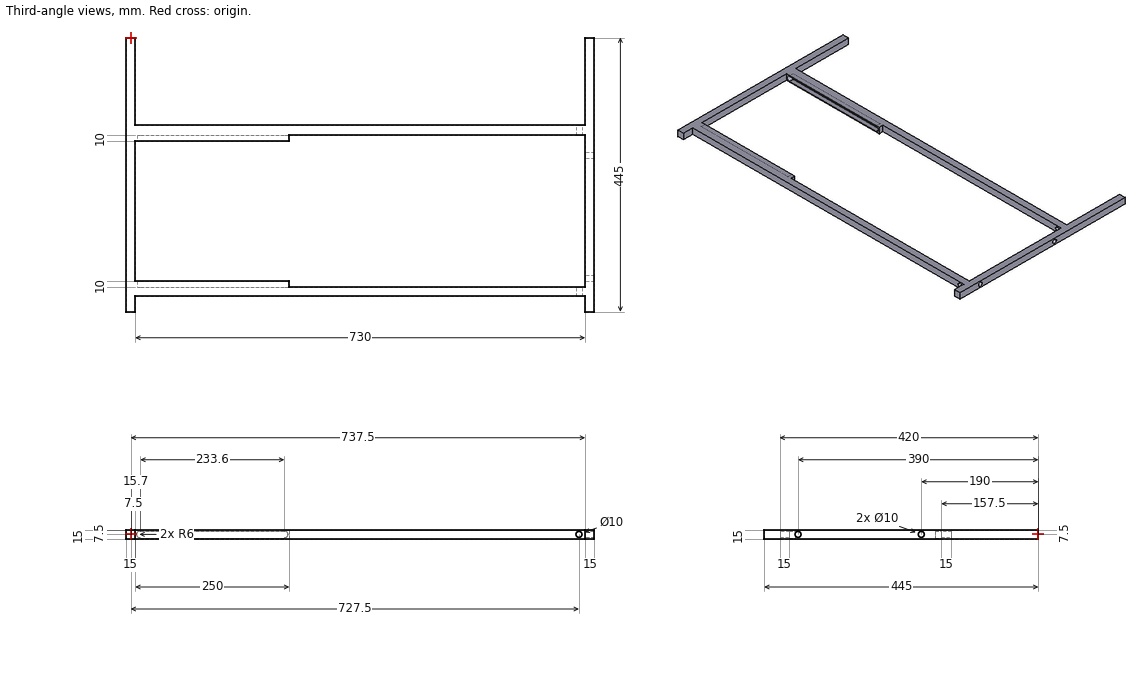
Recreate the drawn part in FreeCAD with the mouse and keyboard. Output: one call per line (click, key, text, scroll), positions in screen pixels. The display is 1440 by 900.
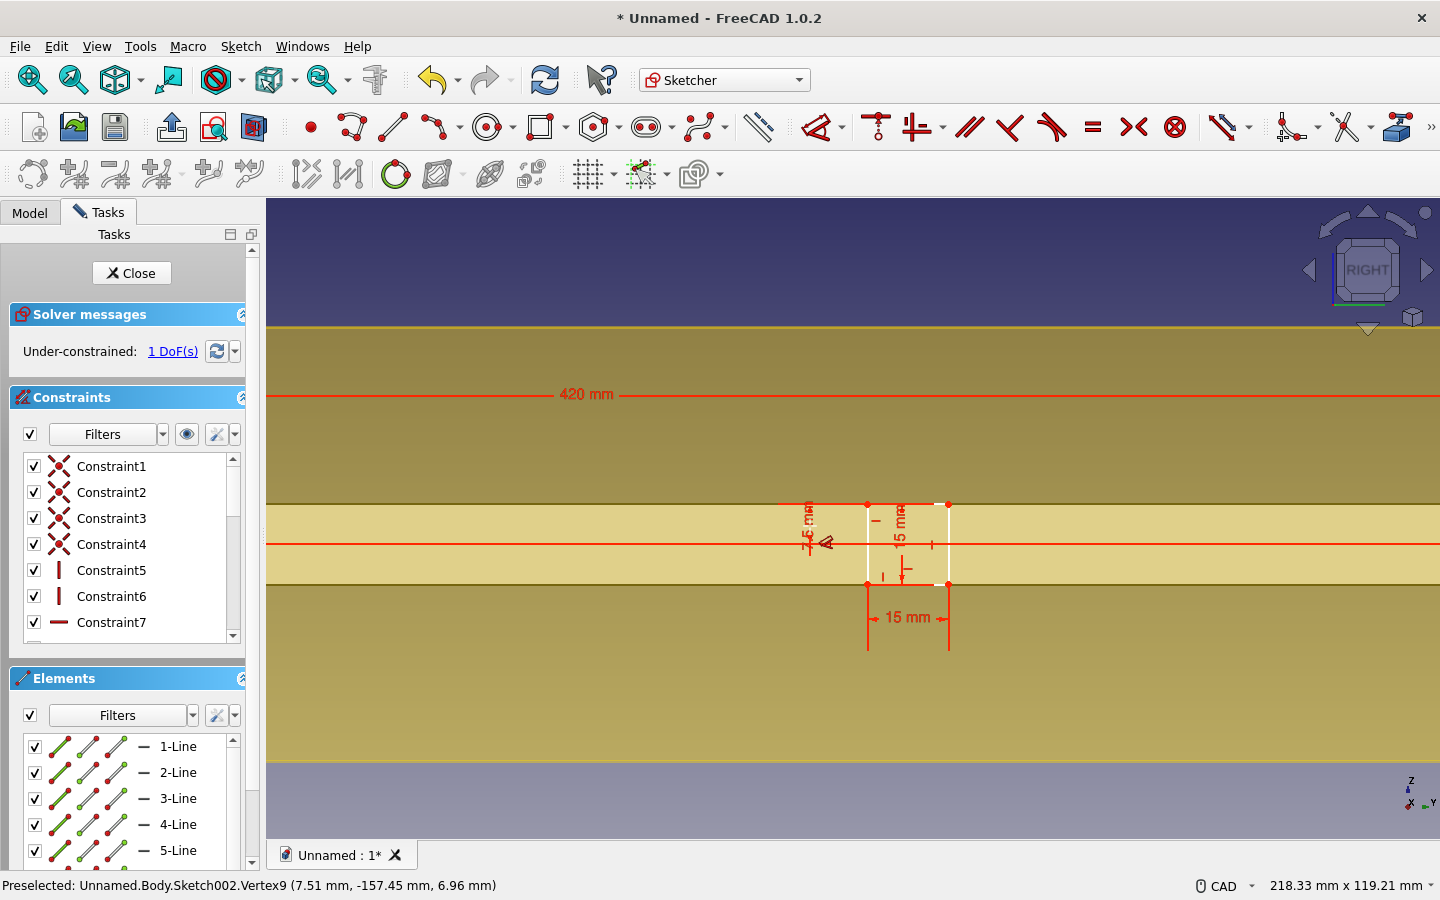
click(868, 504)
click(1071, 470)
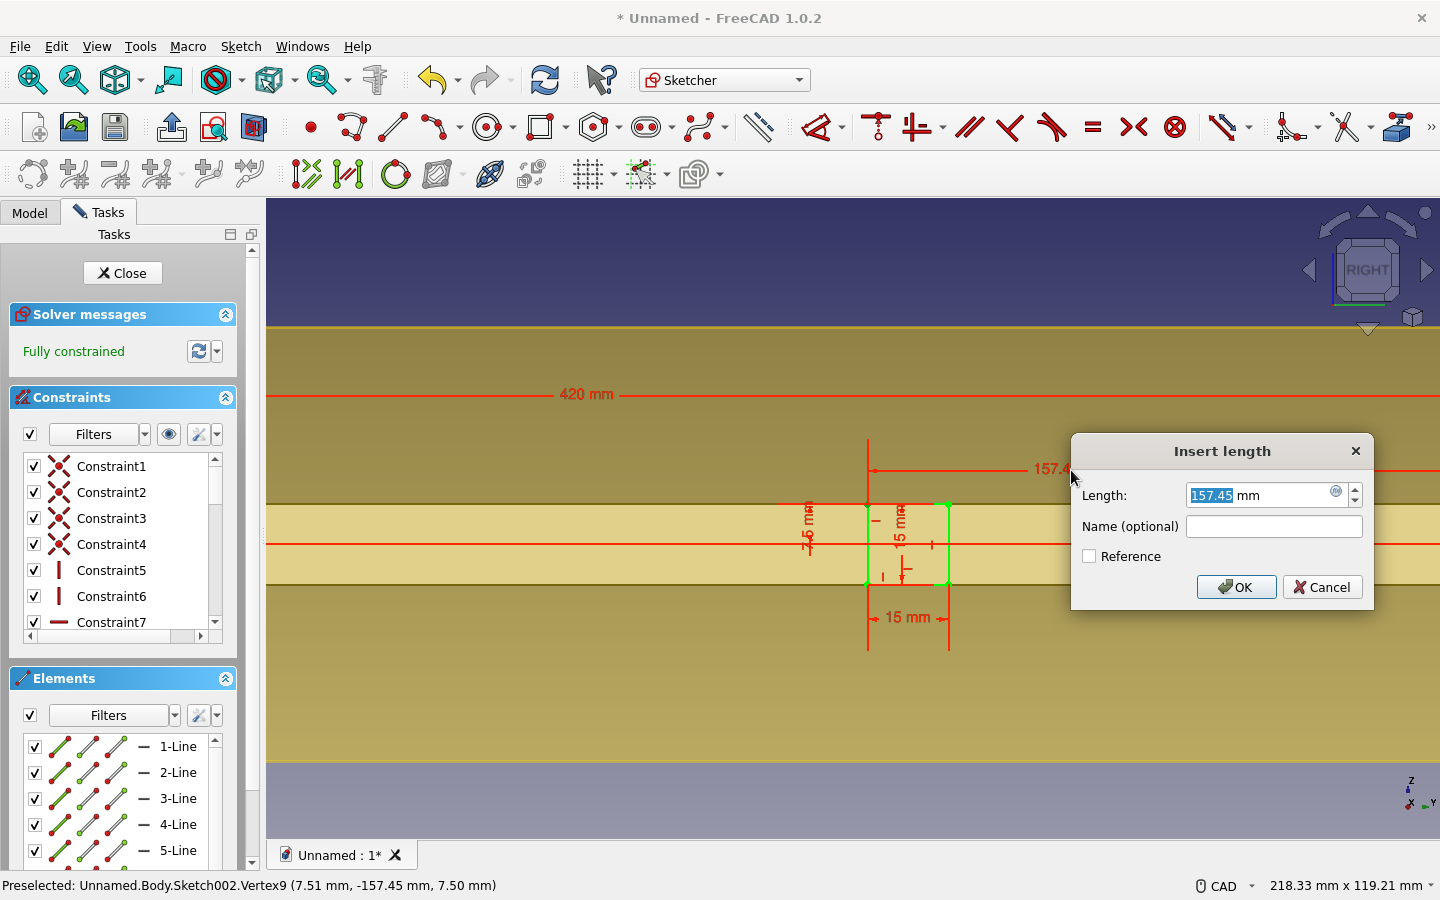
text(157.5)
key(Return)
key(Escape)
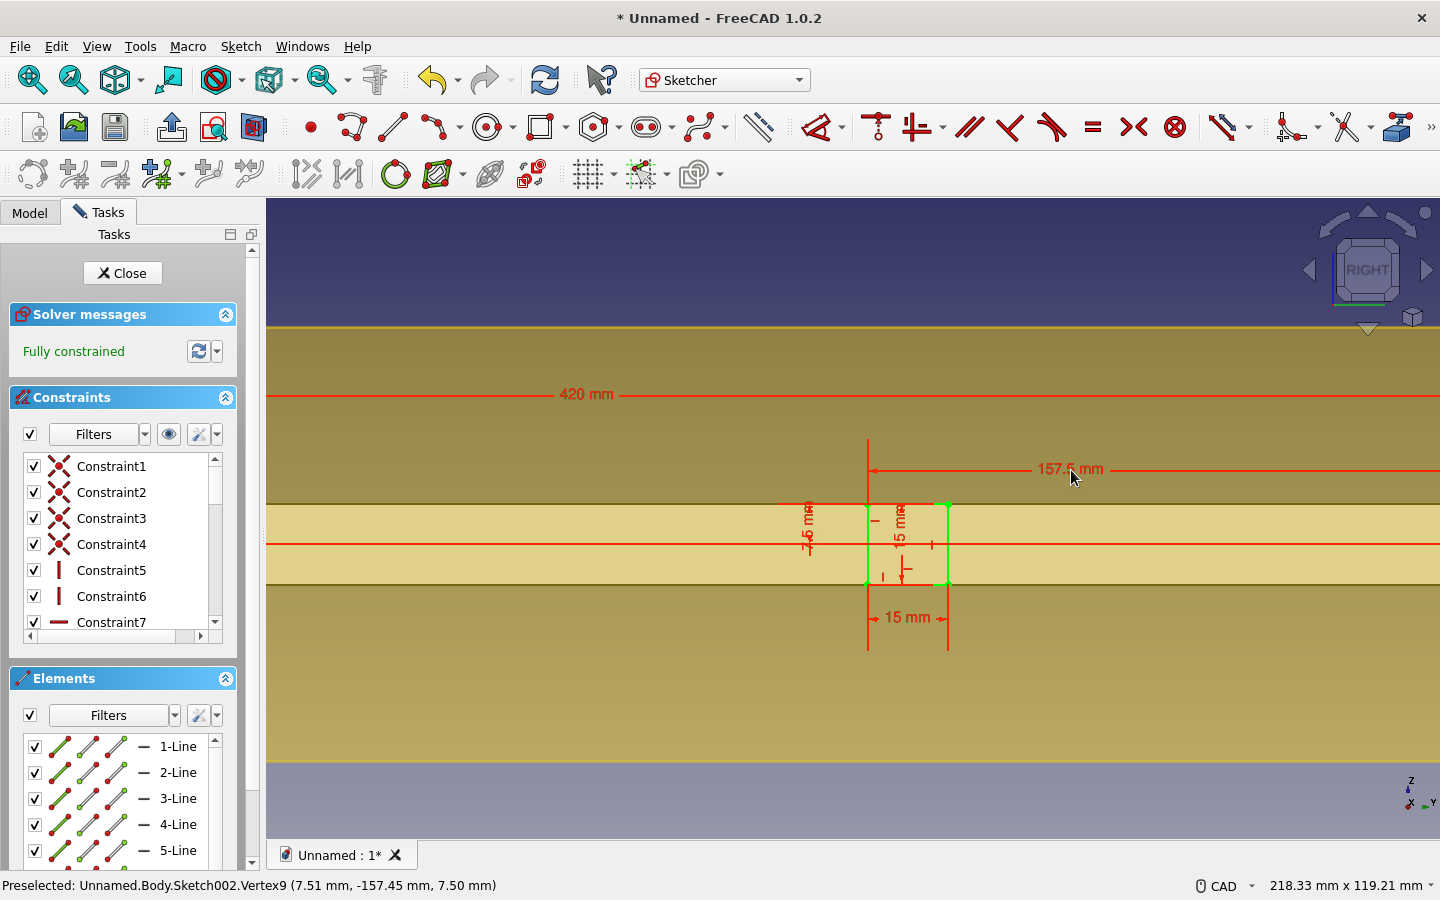
click(123, 273)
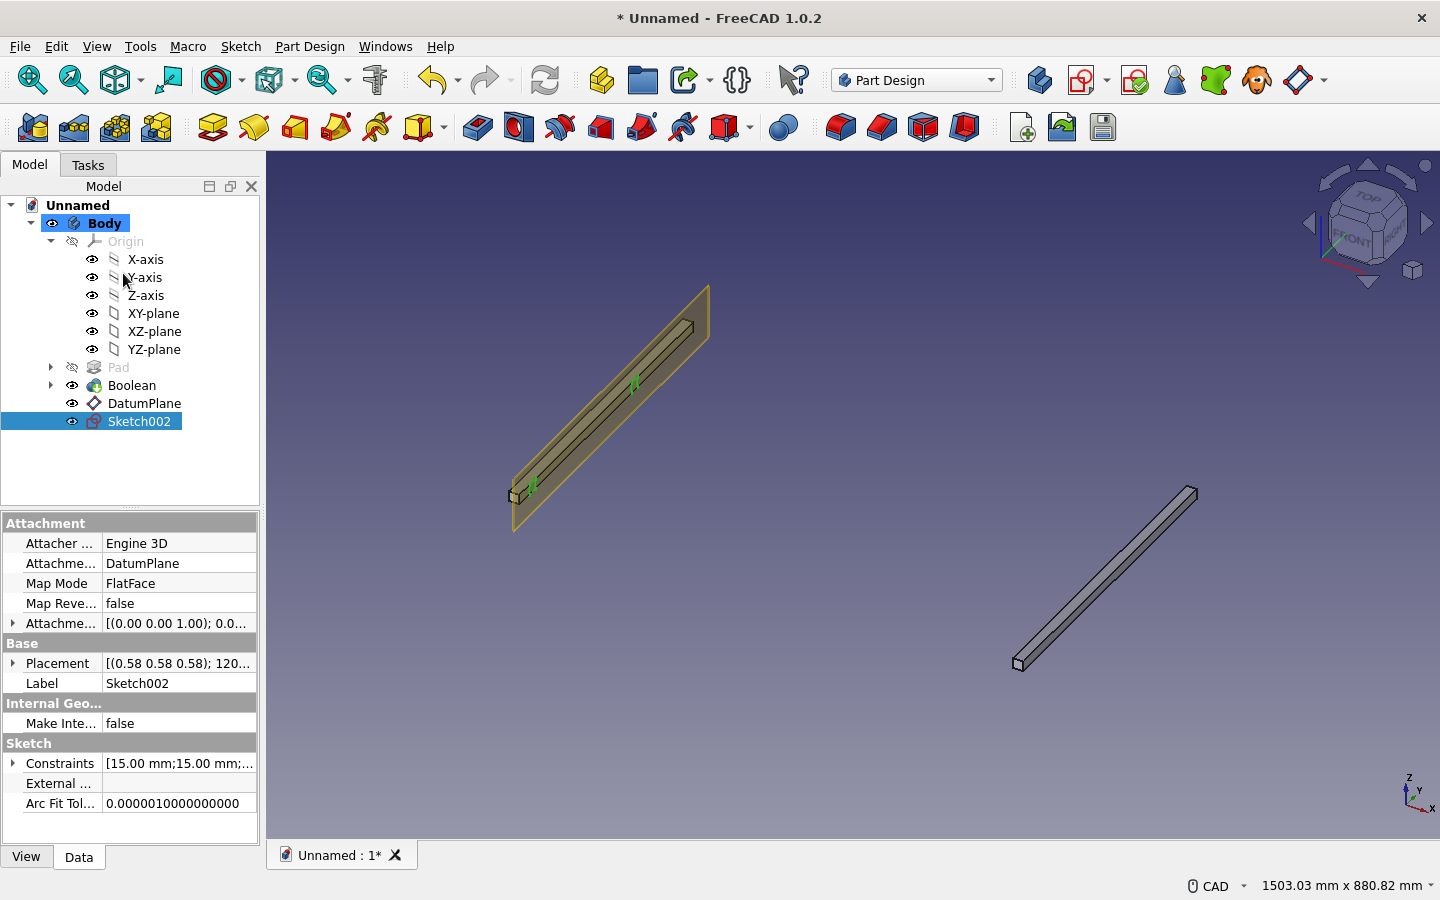
click(213, 128)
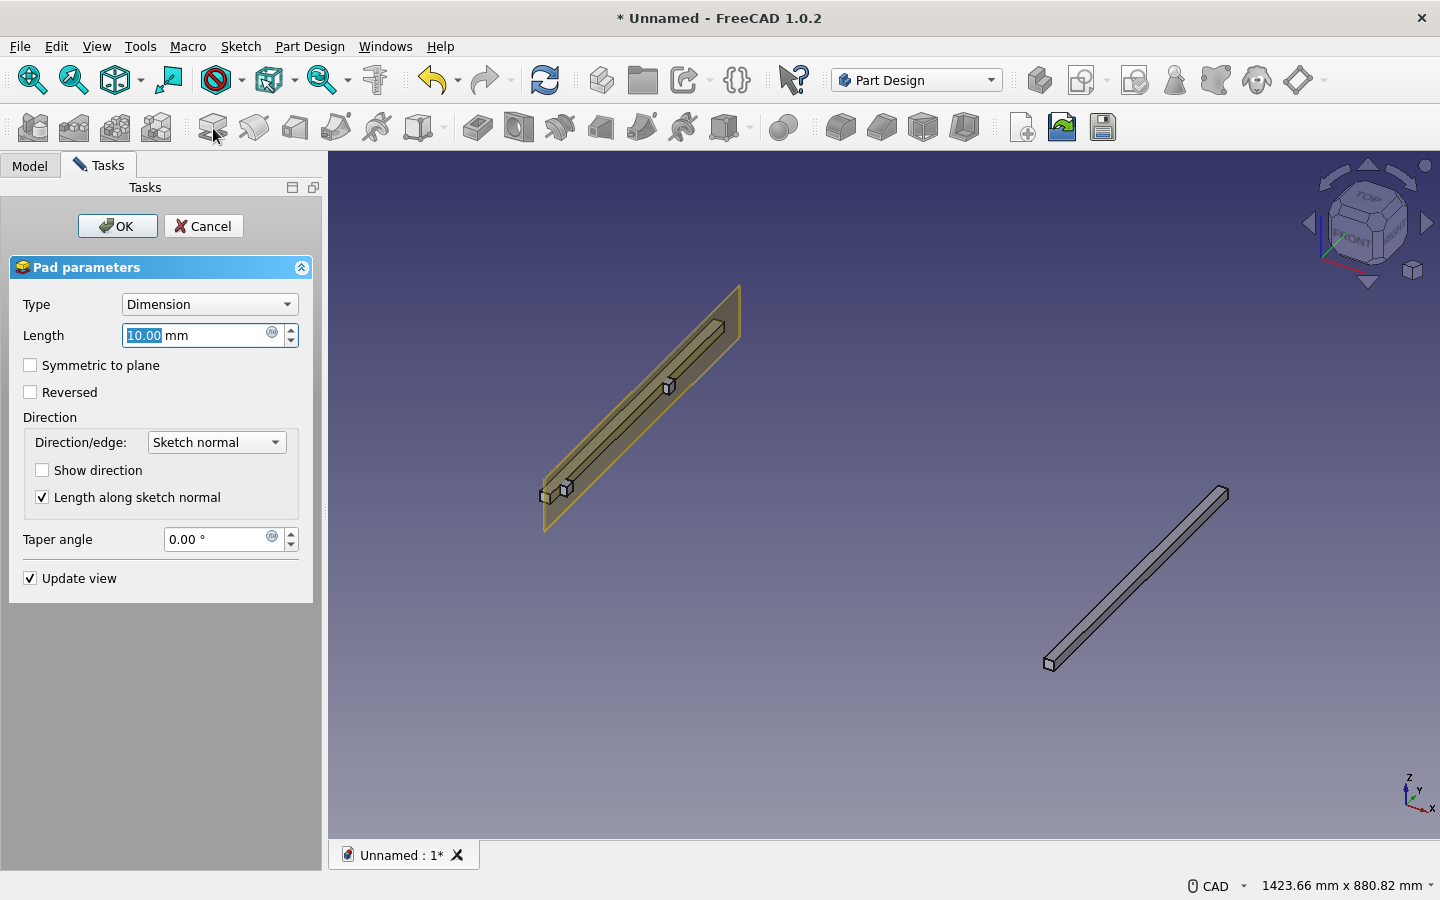
text(730)
key(Tab)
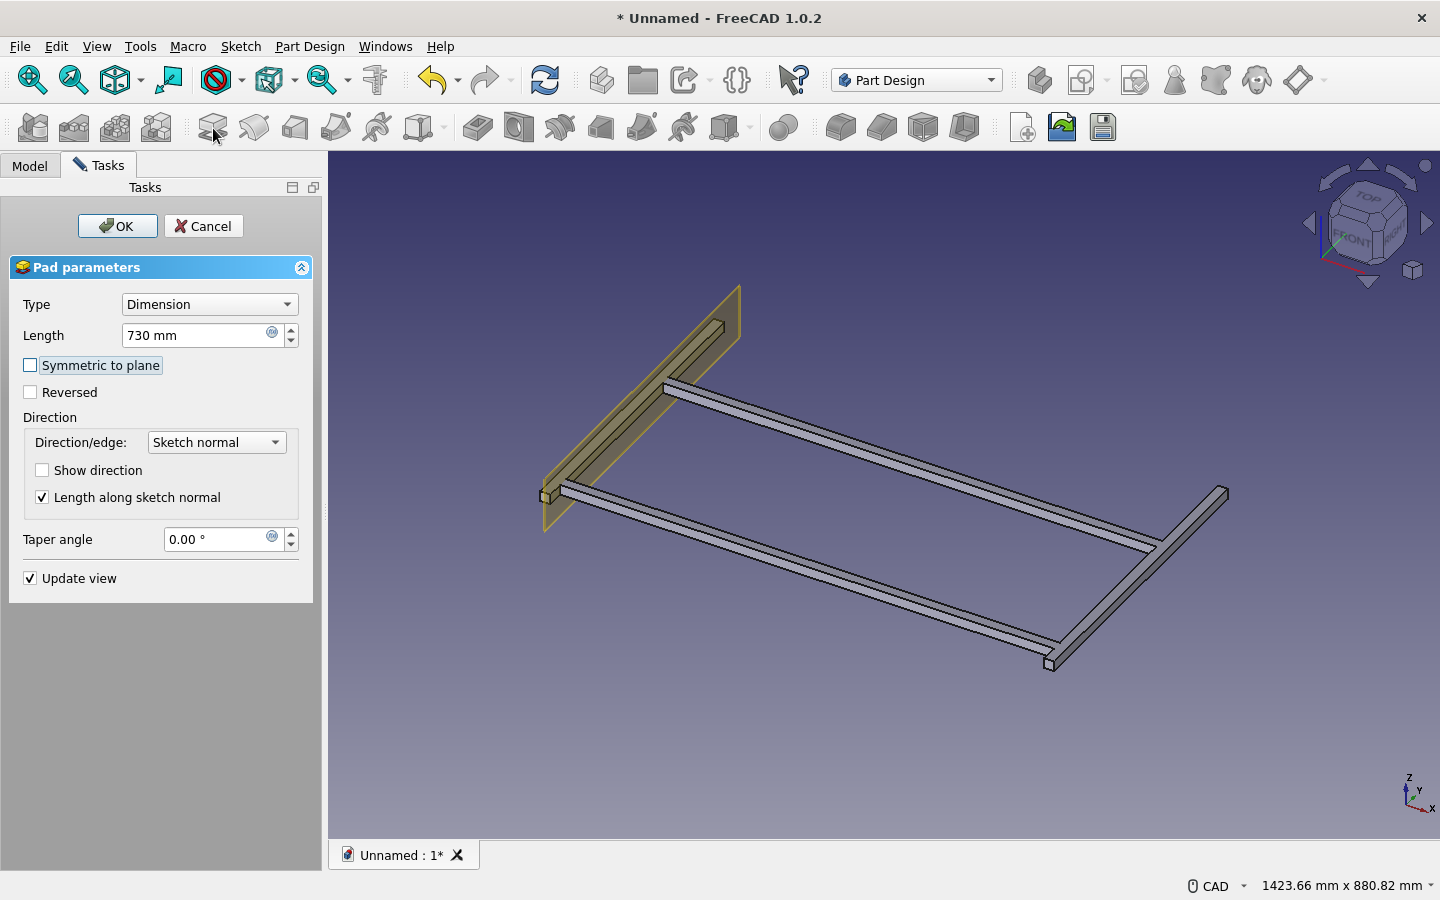
click(118, 226)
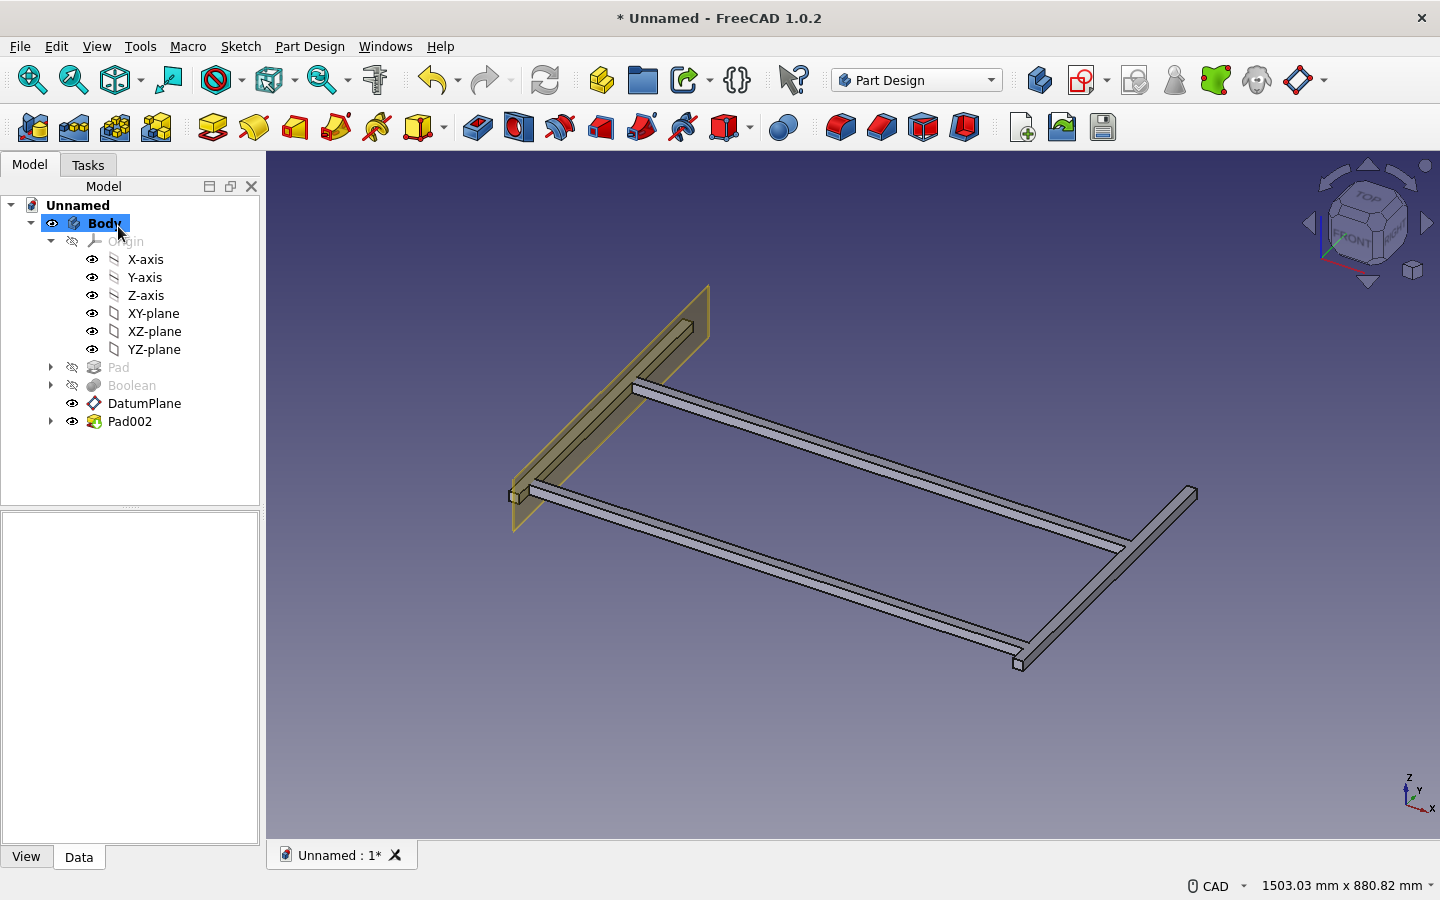
click(117, 403)
key(space)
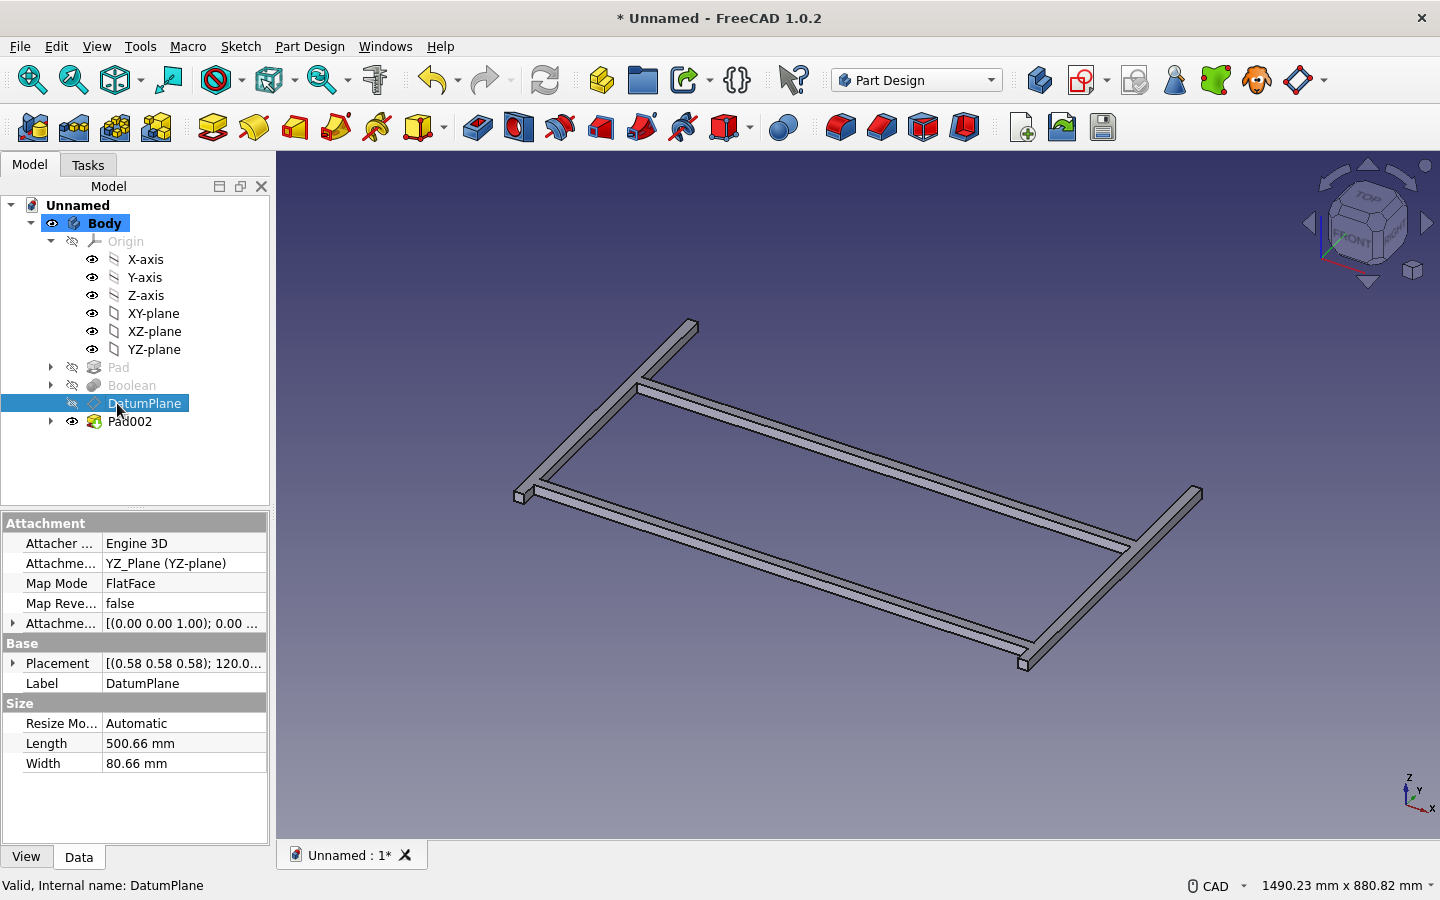
click(137, 349)